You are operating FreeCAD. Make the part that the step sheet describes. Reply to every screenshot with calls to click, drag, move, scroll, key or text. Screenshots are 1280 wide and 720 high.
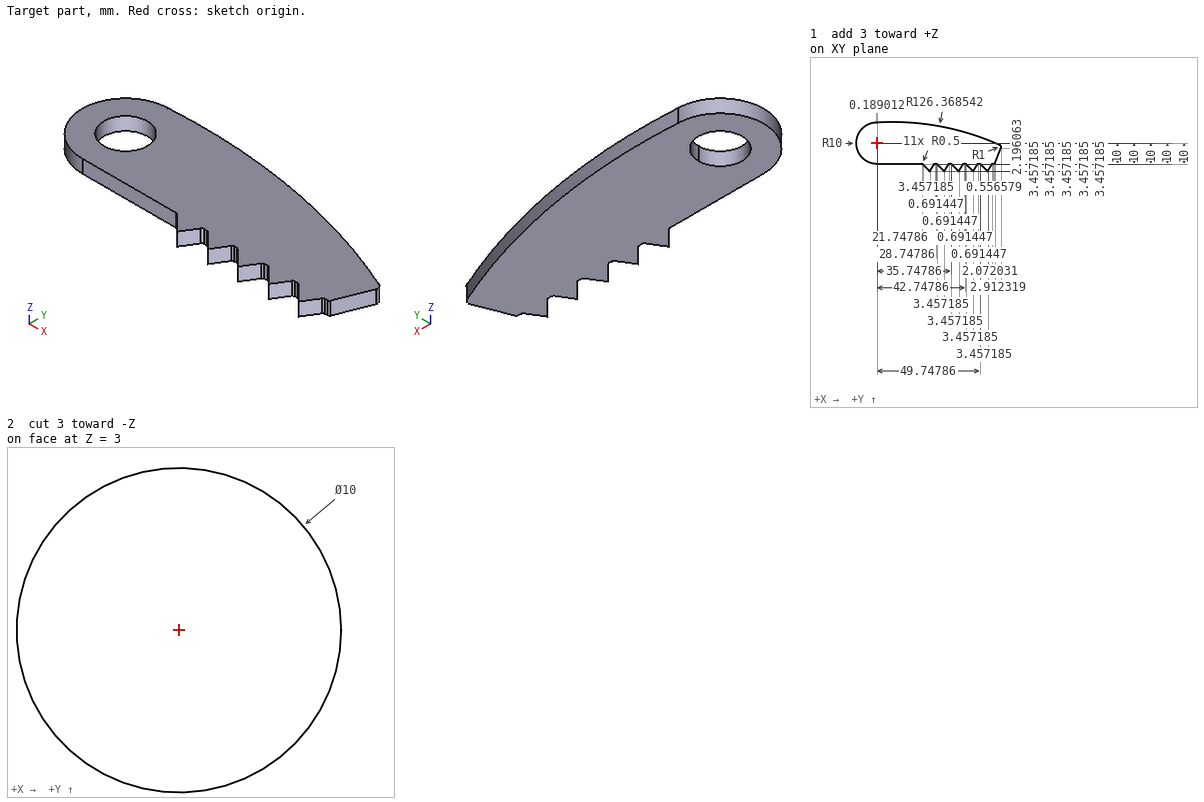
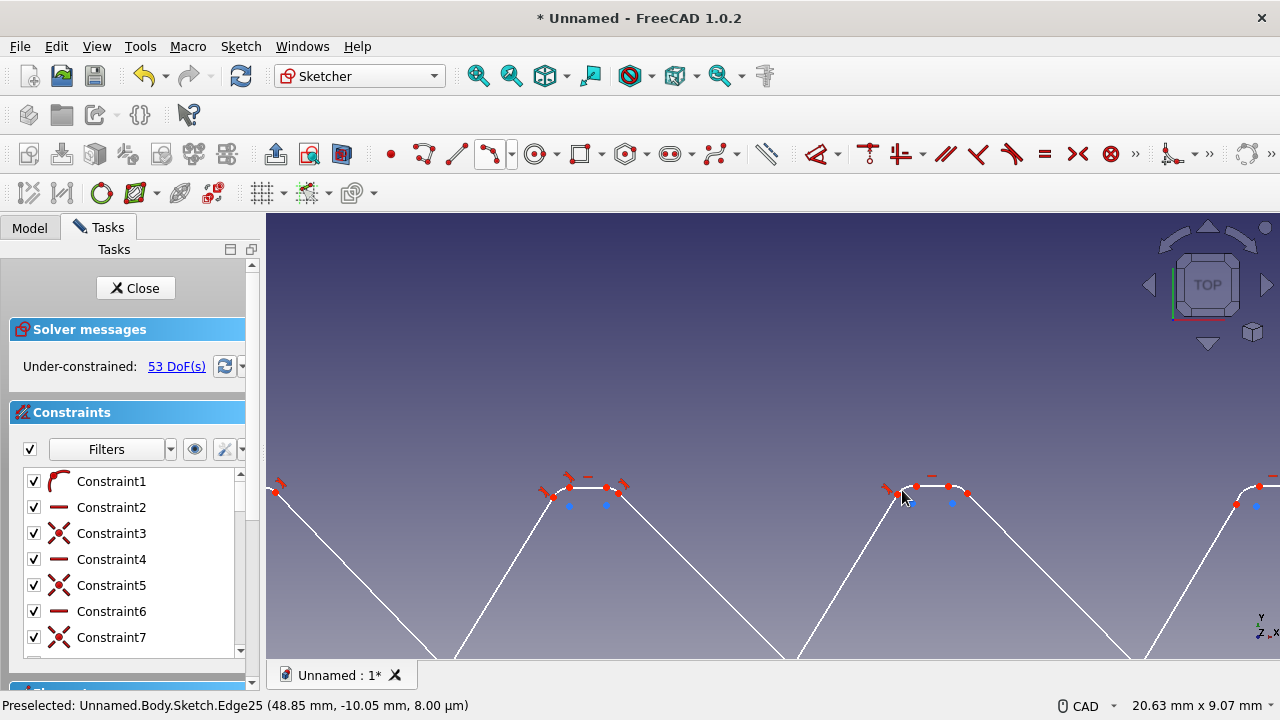
scroll(926, 486, up, 2)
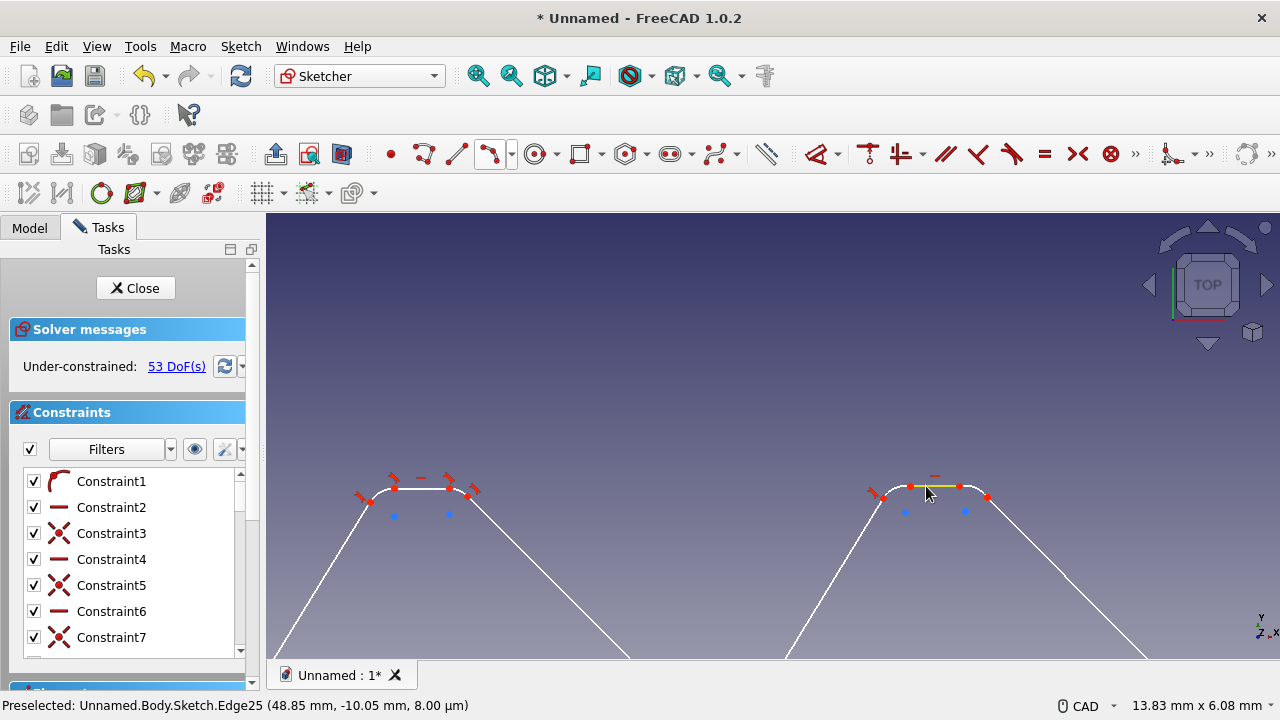
click(926, 486)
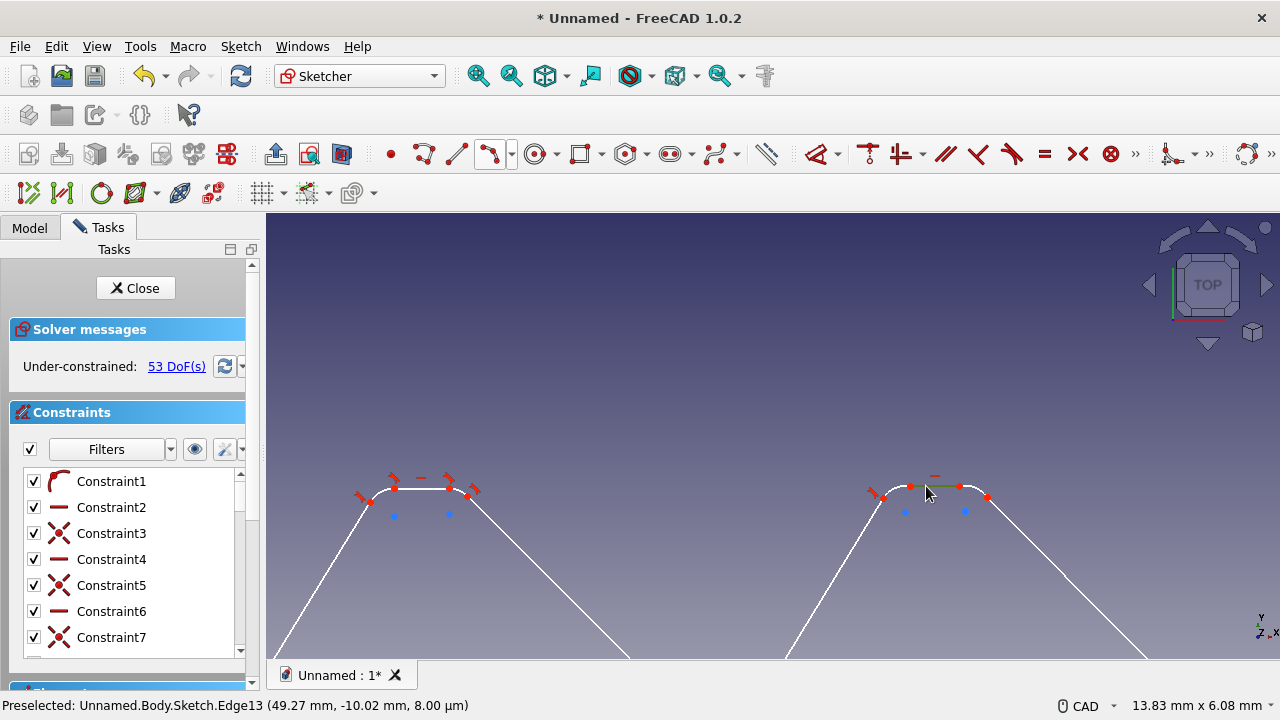
scroll(901, 486, up, 2)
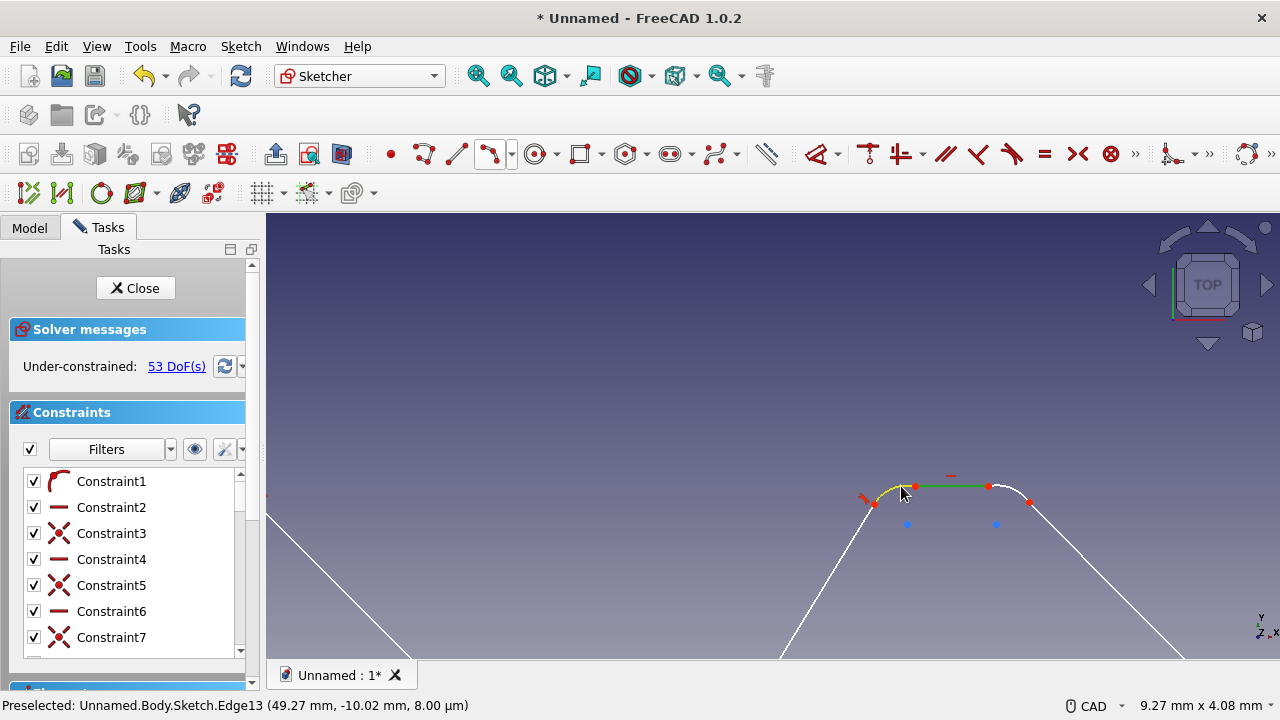
click(901, 486)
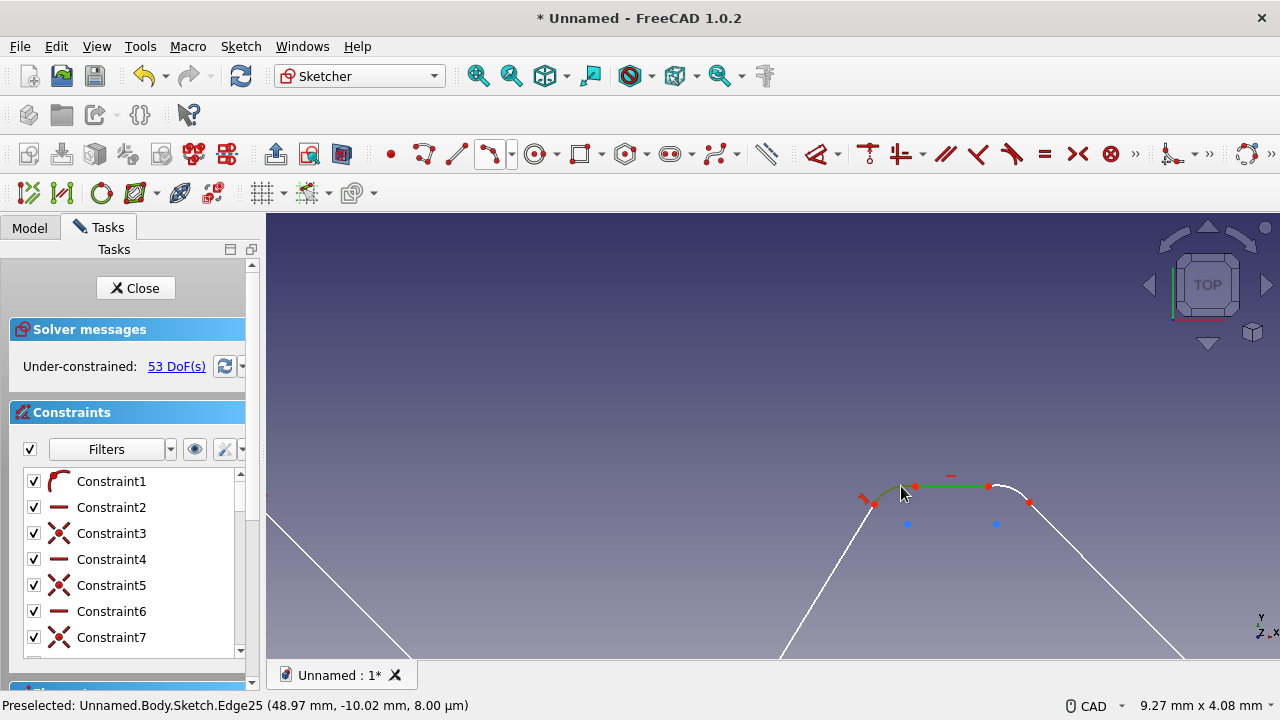
click(1012, 154)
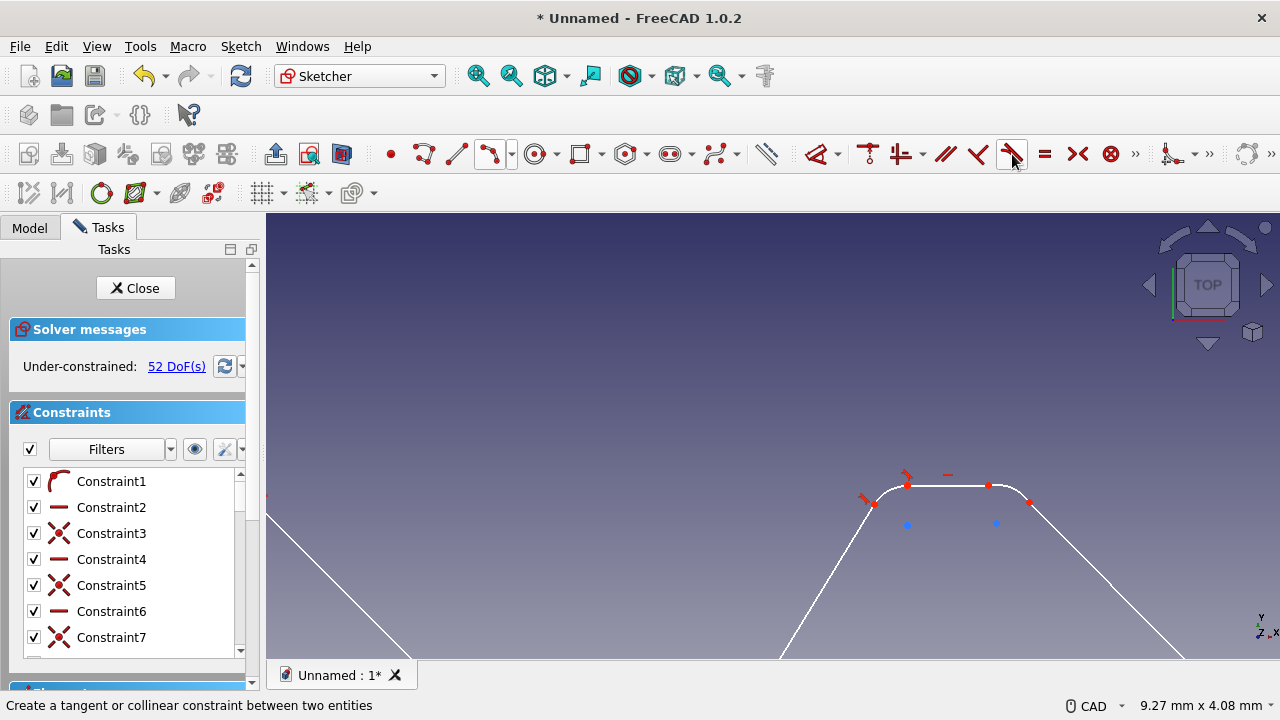
click(932, 486)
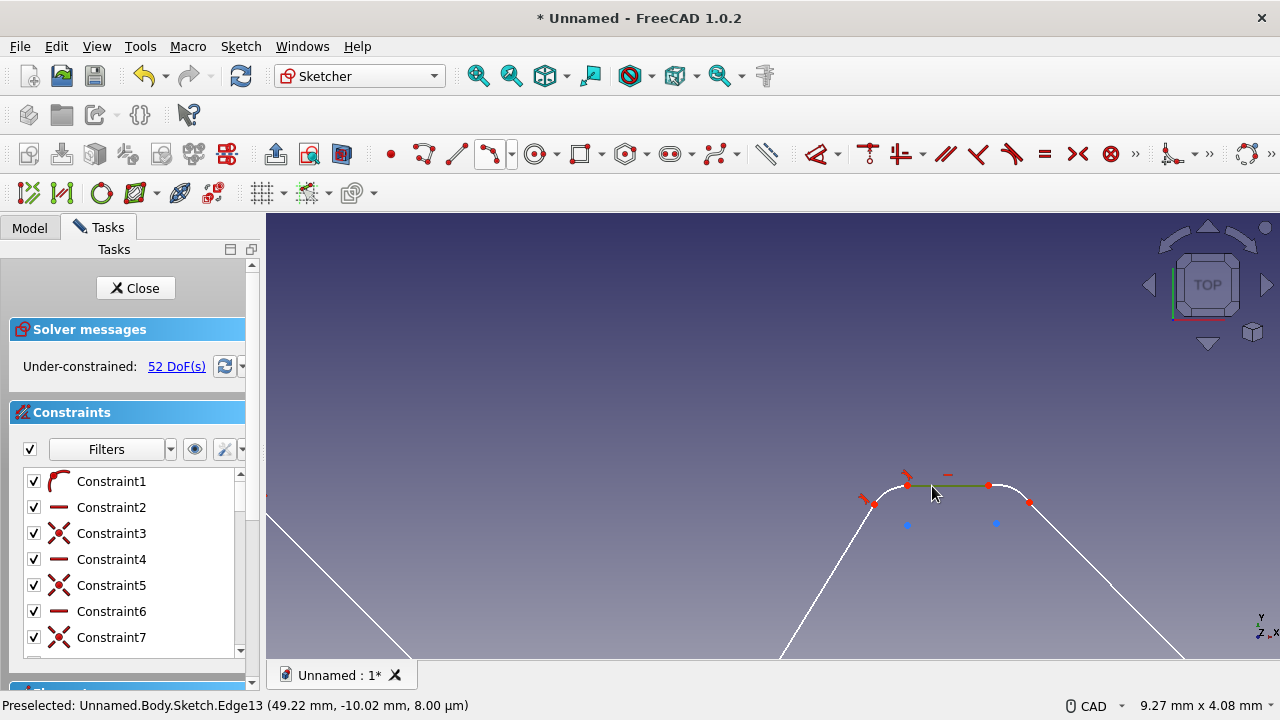
click(1019, 492)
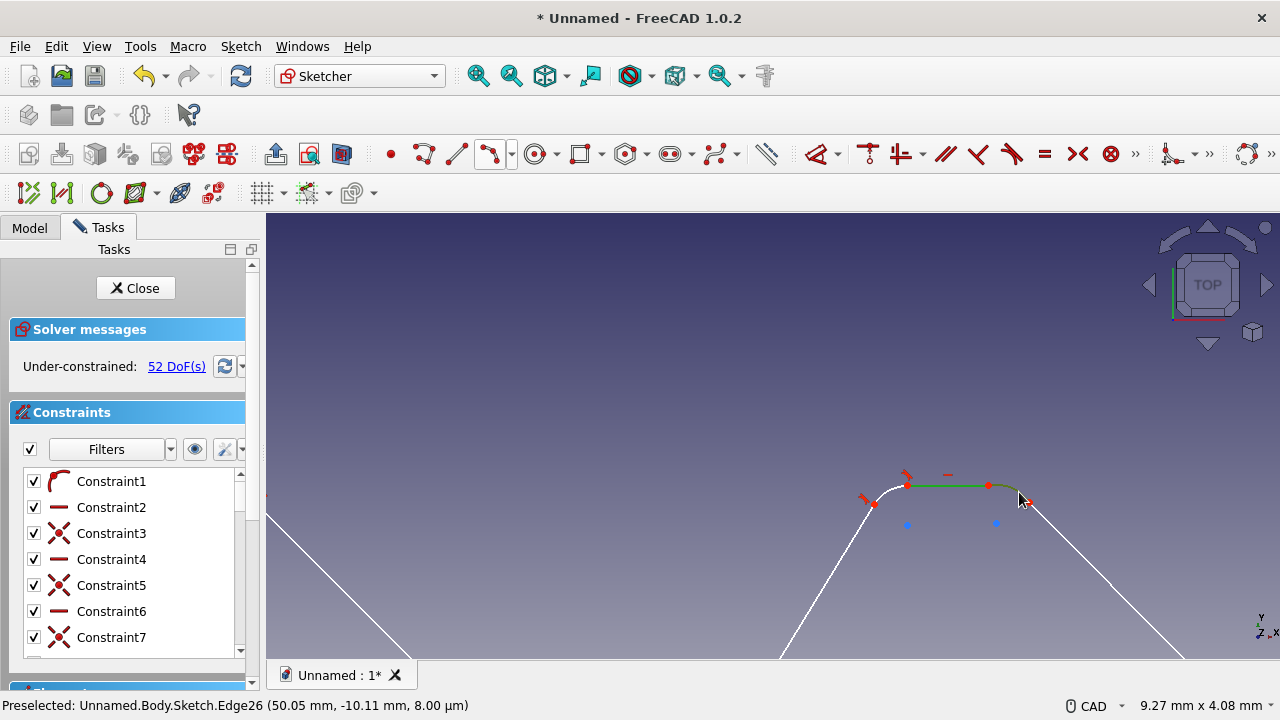
click(1012, 154)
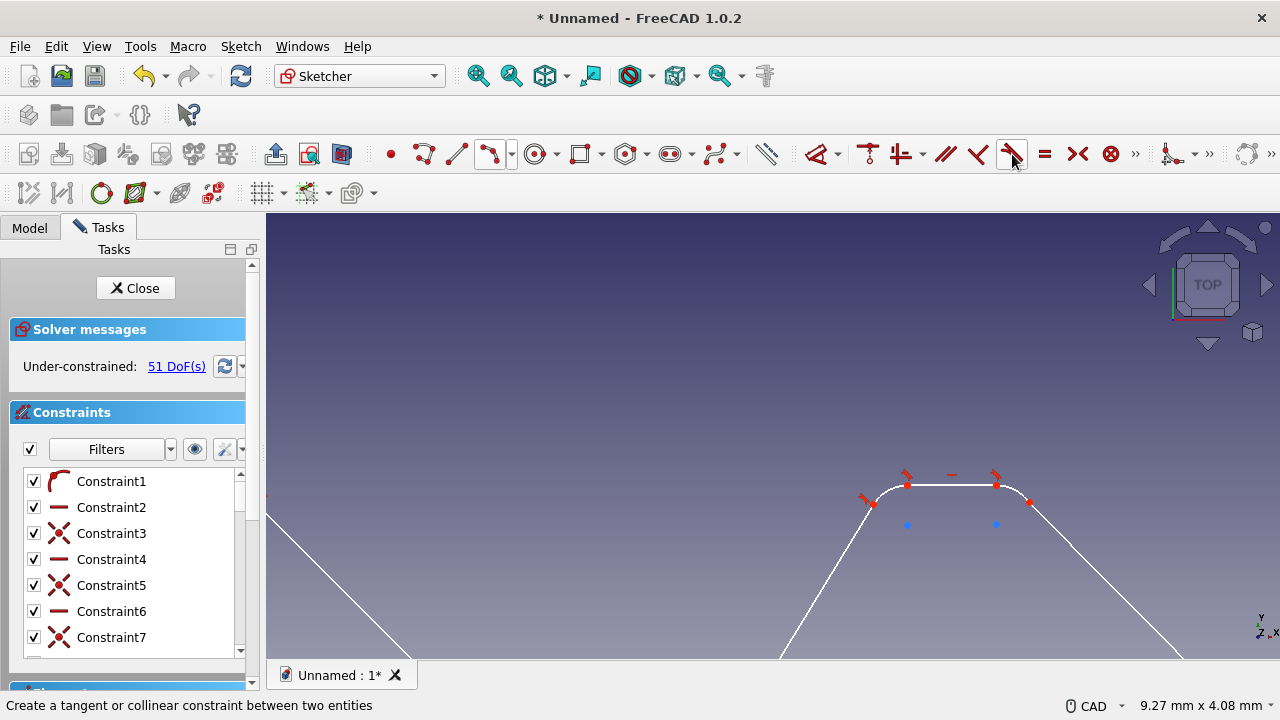
scroll(899, 504, down, 13)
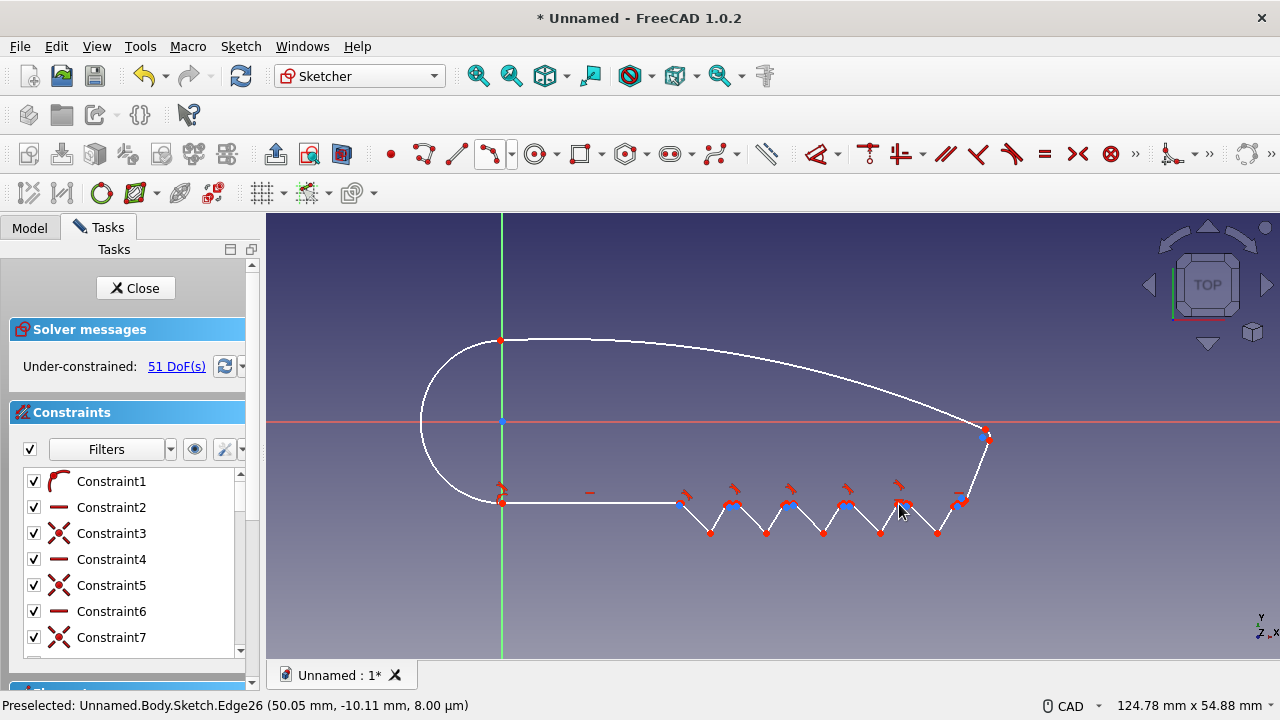
scroll(915, 510, up, 3)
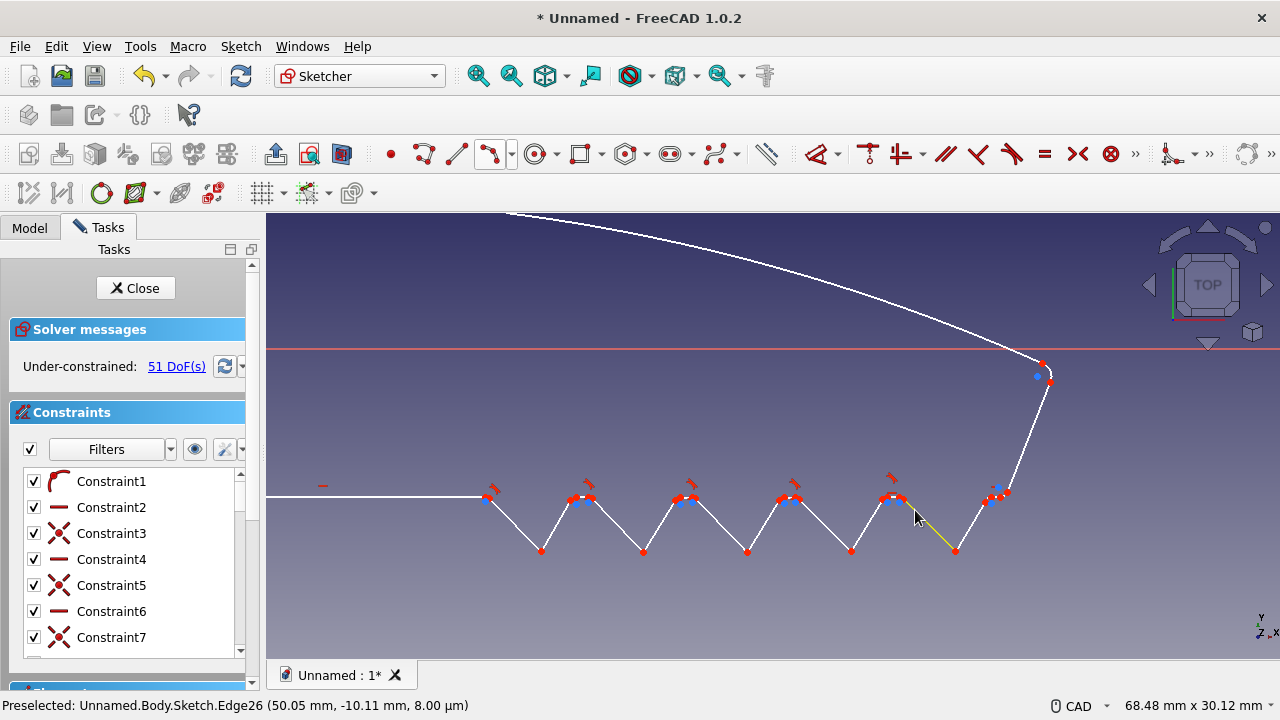
click(914, 510)